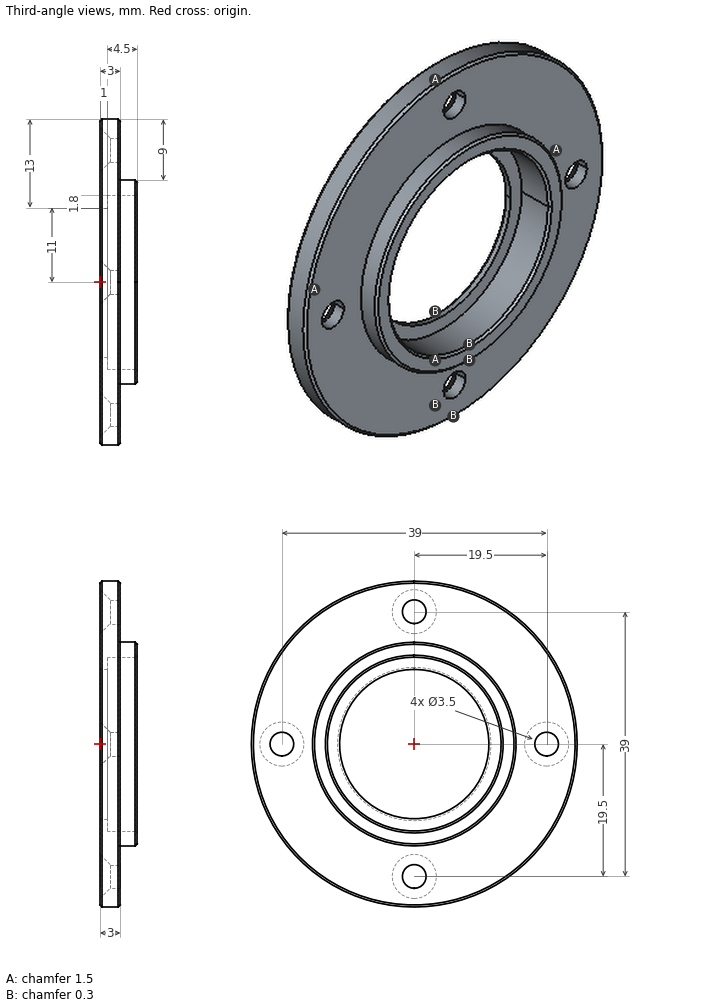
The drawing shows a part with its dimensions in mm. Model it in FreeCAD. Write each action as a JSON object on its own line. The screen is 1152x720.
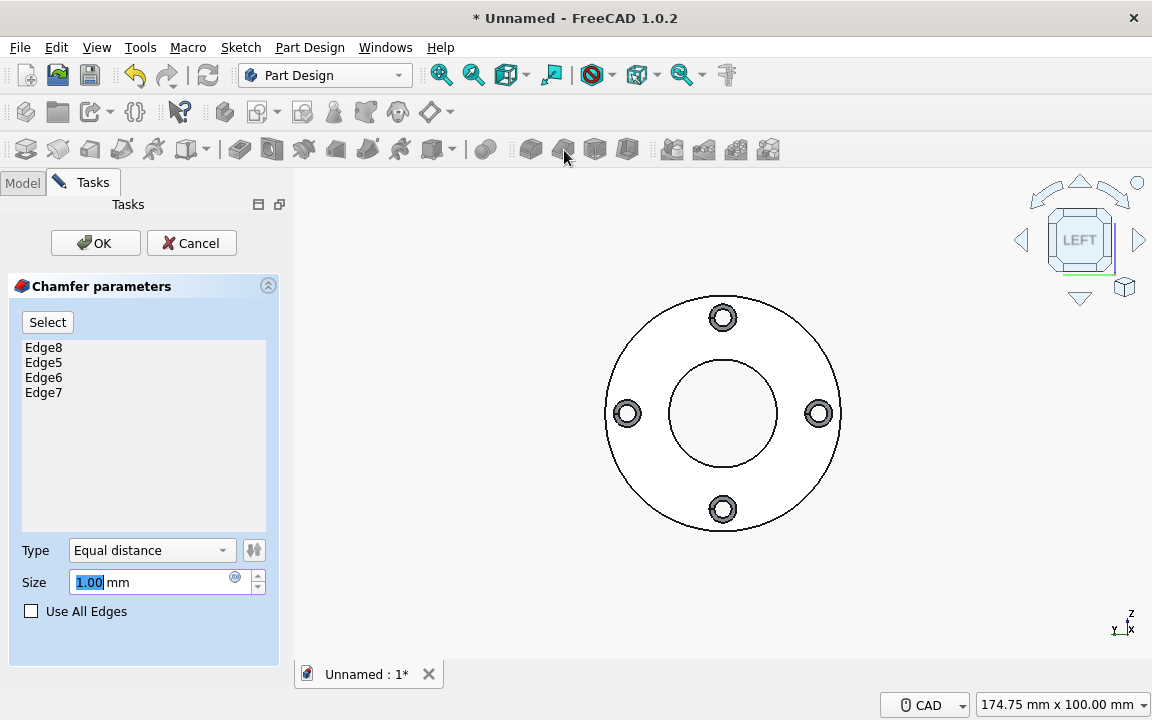
{"action": "type", "text": "1.5"}
{"action": "key", "text": "Tab"}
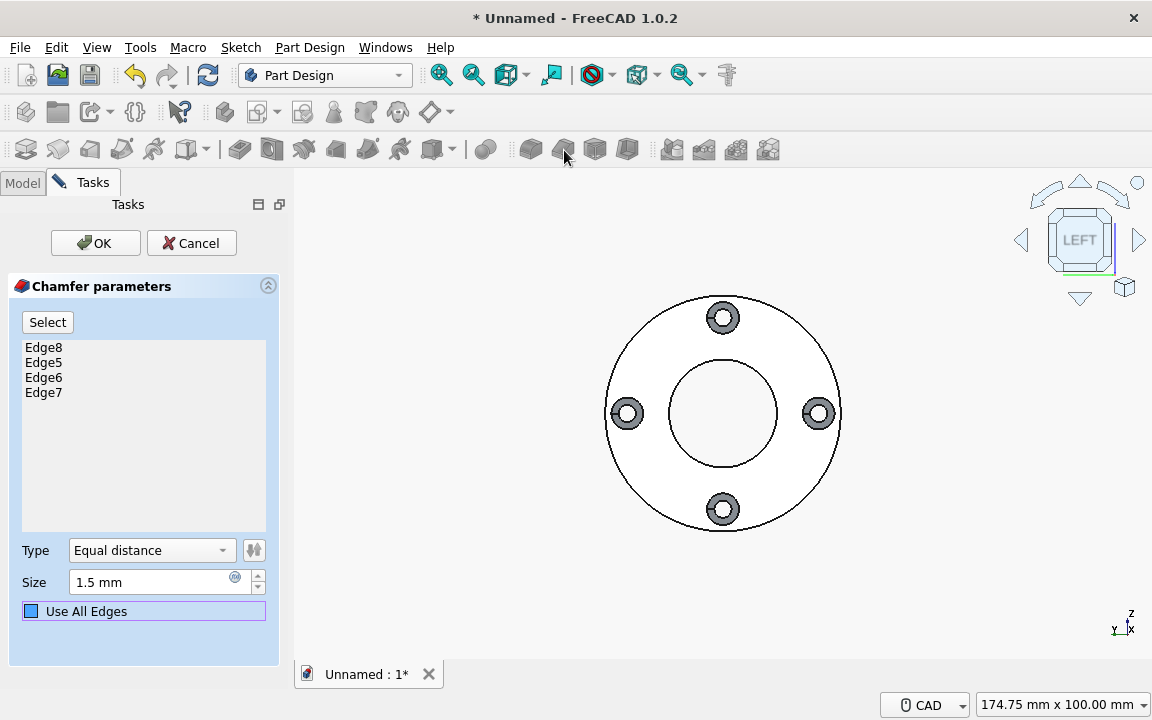
{"action": "left_click", "coordinate": [96, 243]}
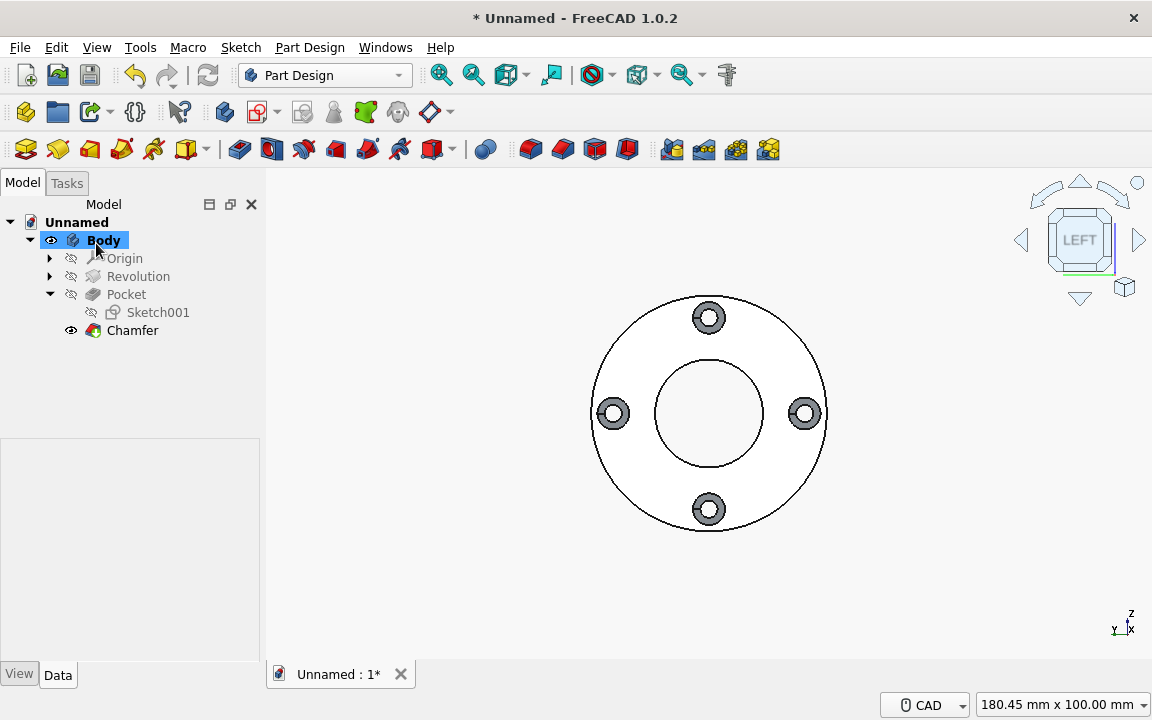
{"action": "left_click", "coordinate": [827, 412]}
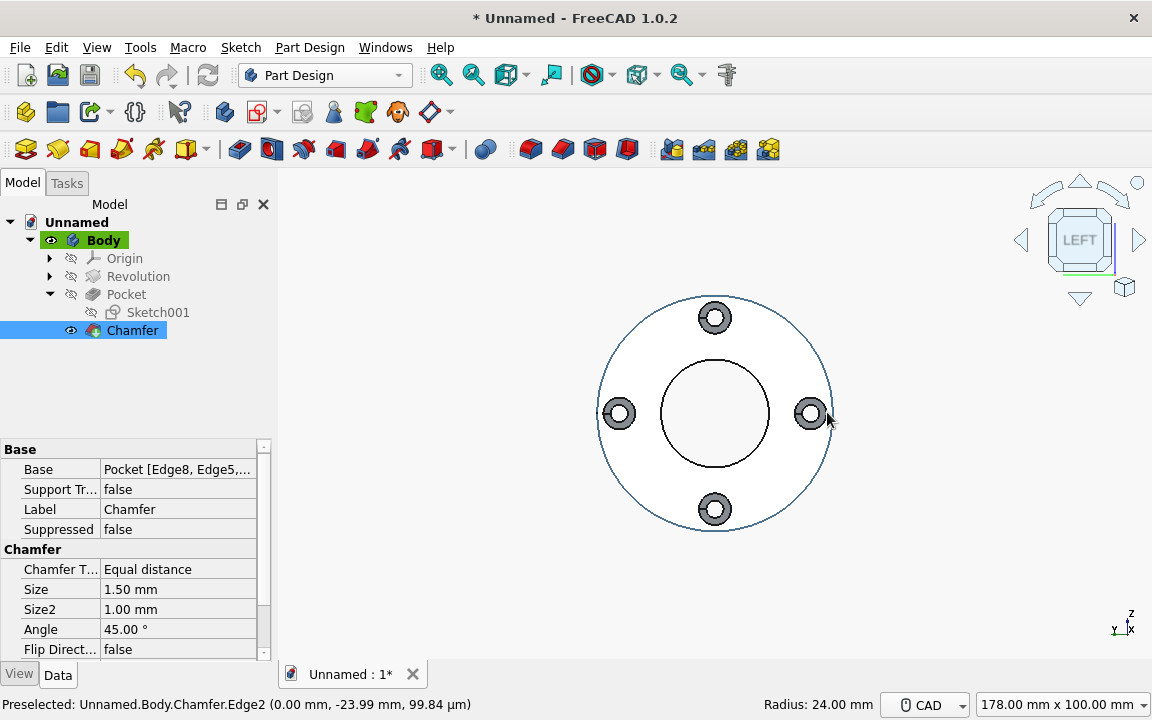
{"action": "left_click", "coordinate": [759, 381], "text": "ctrl"}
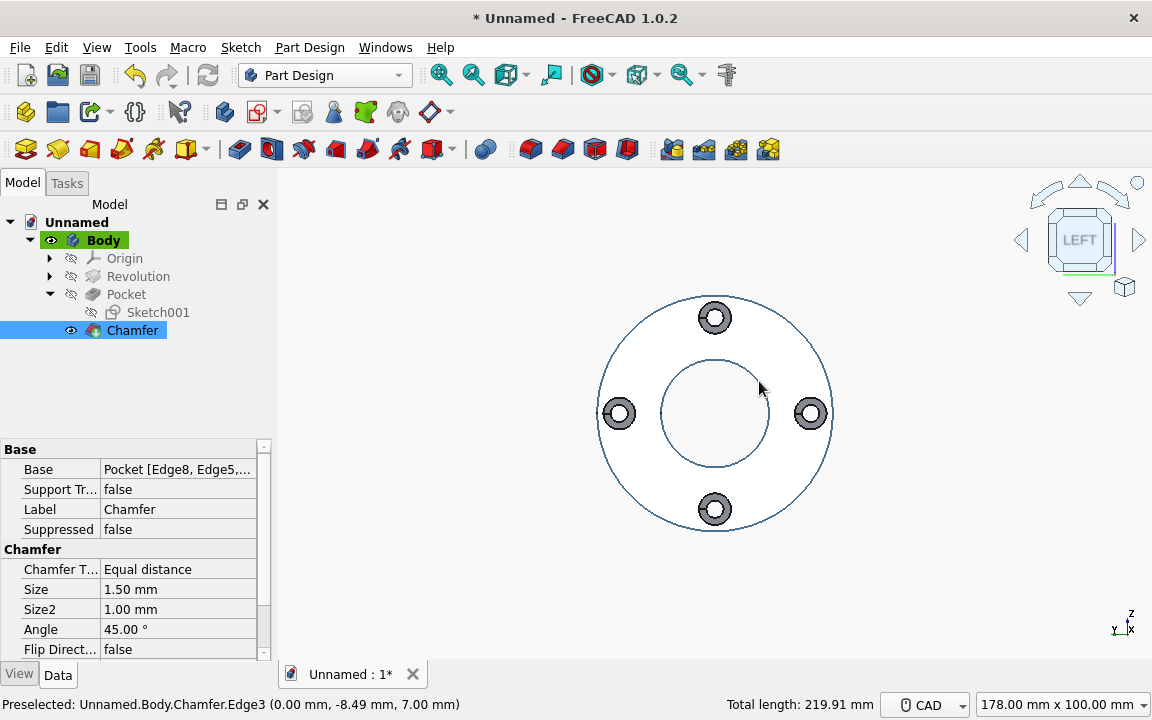
{"action": "key", "text": "0"}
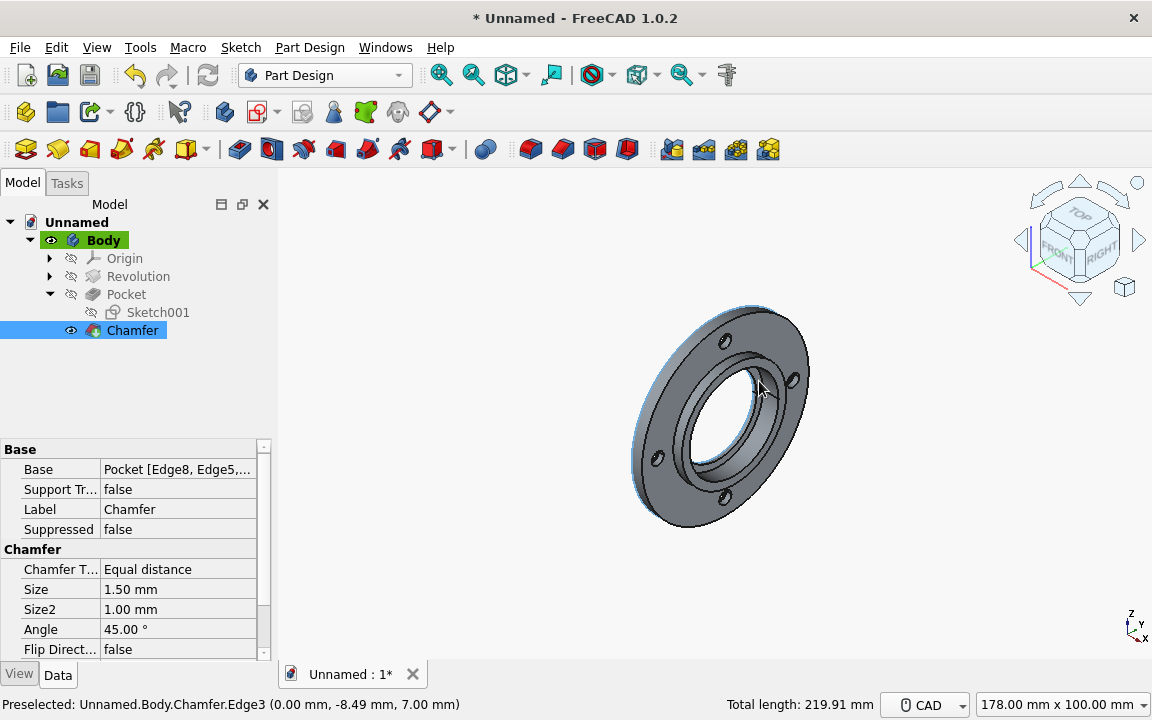
{"action": "left_click", "coordinate": [642, 467], "text": "ctrl"}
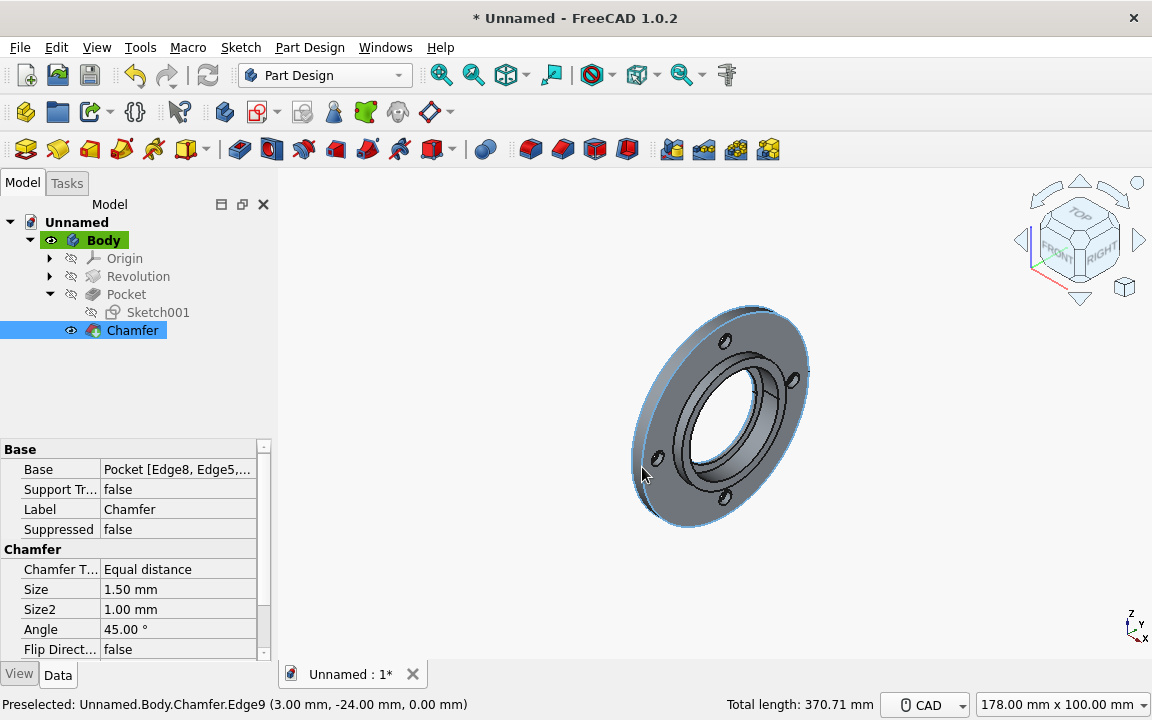
{"action": "left_click", "coordinate": [698, 474], "text": "ctrl"}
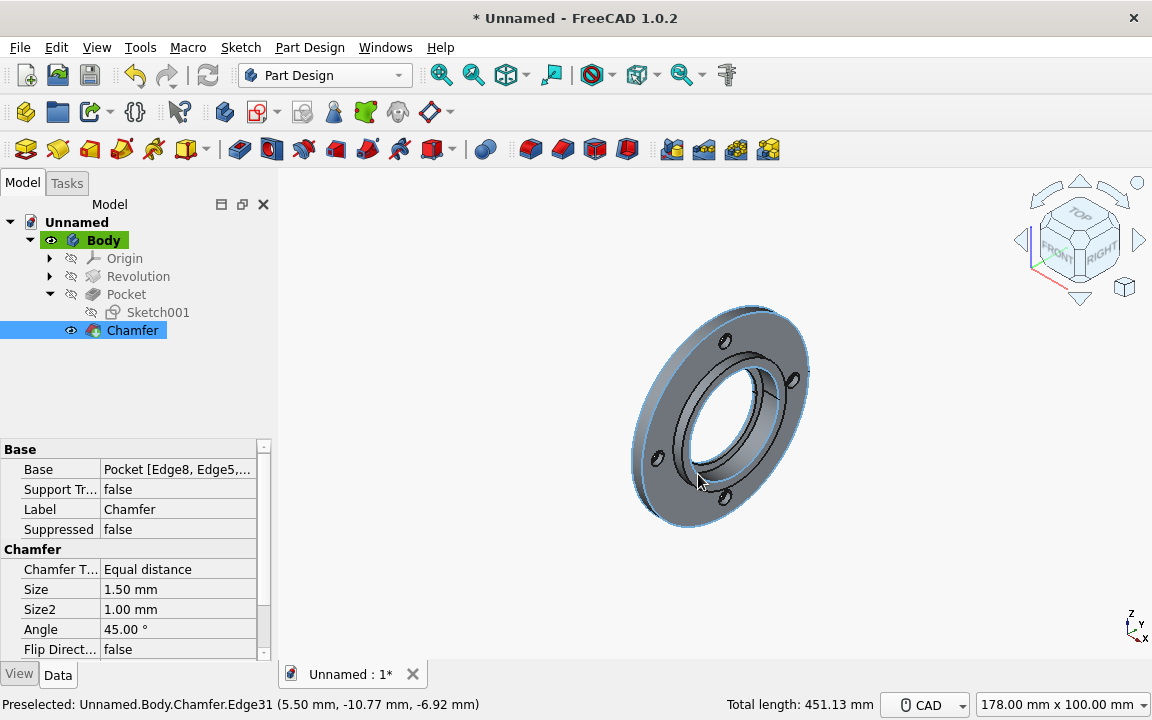
{"action": "left_click", "coordinate": [682, 454], "text": "ctrl"}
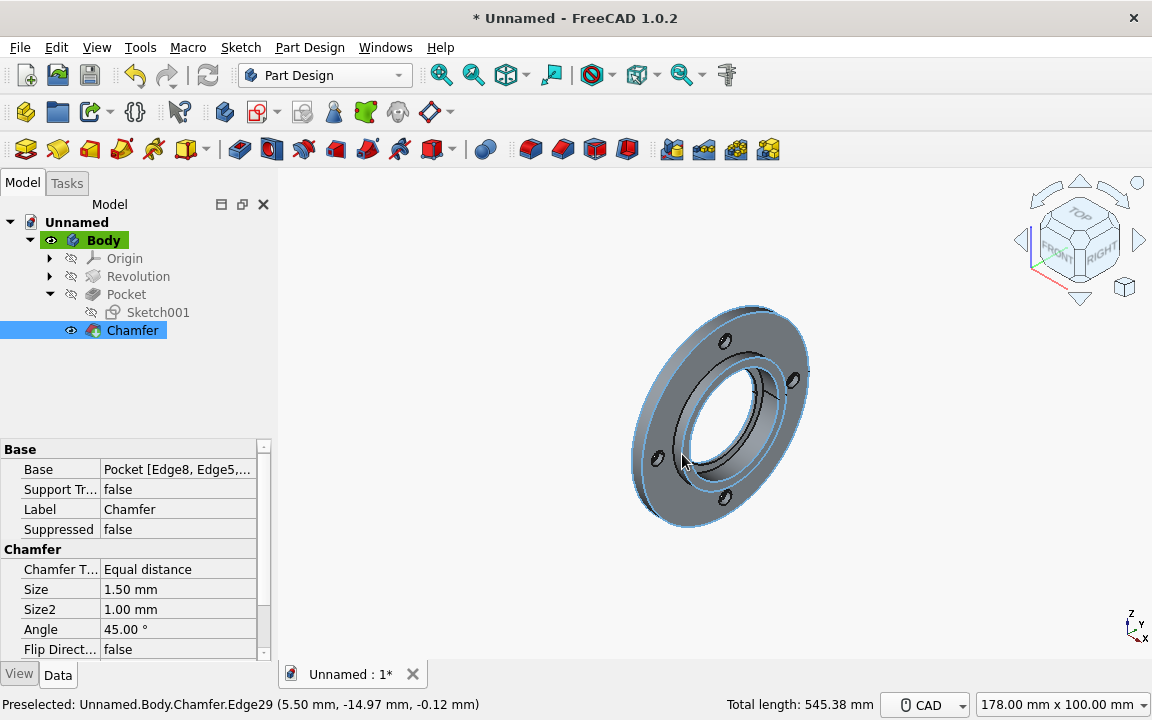
{"action": "left_click", "coordinate": [564, 150]}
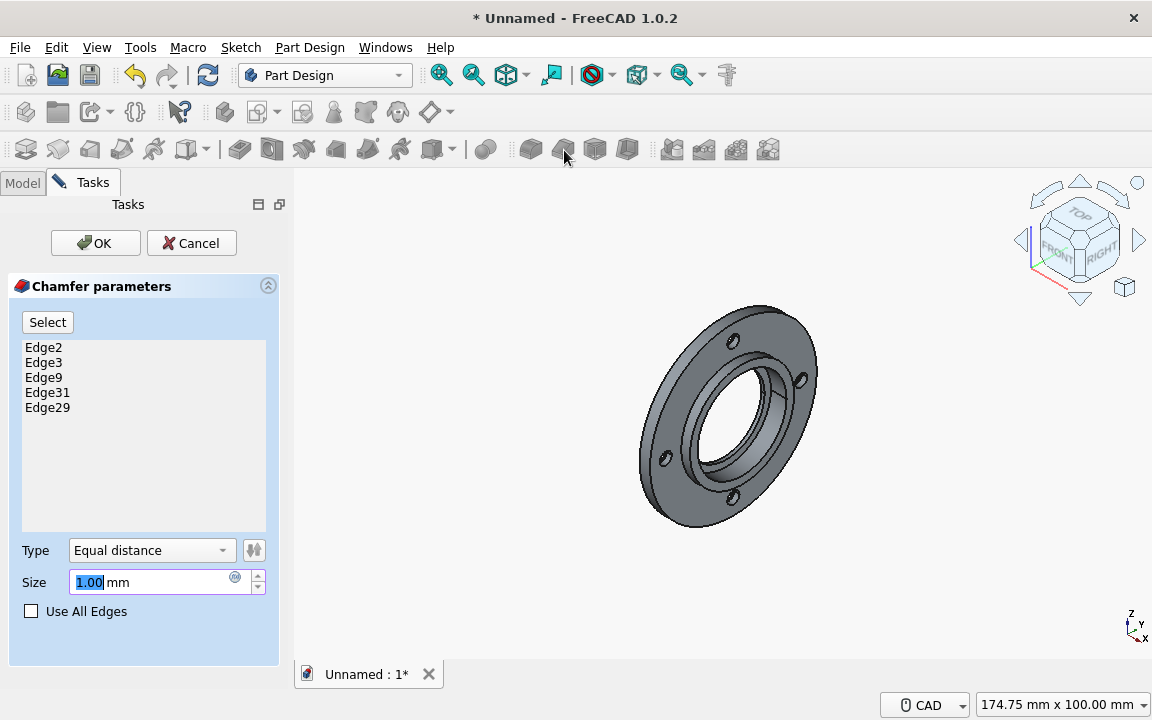
{"action": "type", "text": "0.3"}
{"action": "key", "text": "Tab"}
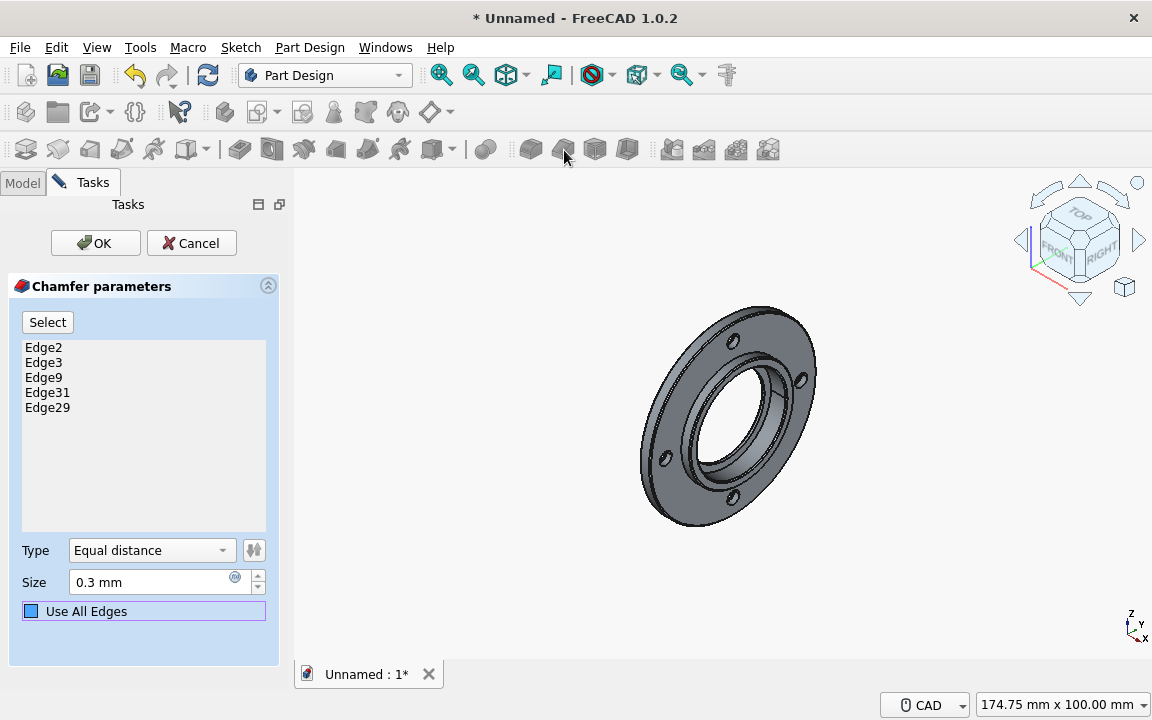
{"action": "left_click", "coordinate": [96, 243]}